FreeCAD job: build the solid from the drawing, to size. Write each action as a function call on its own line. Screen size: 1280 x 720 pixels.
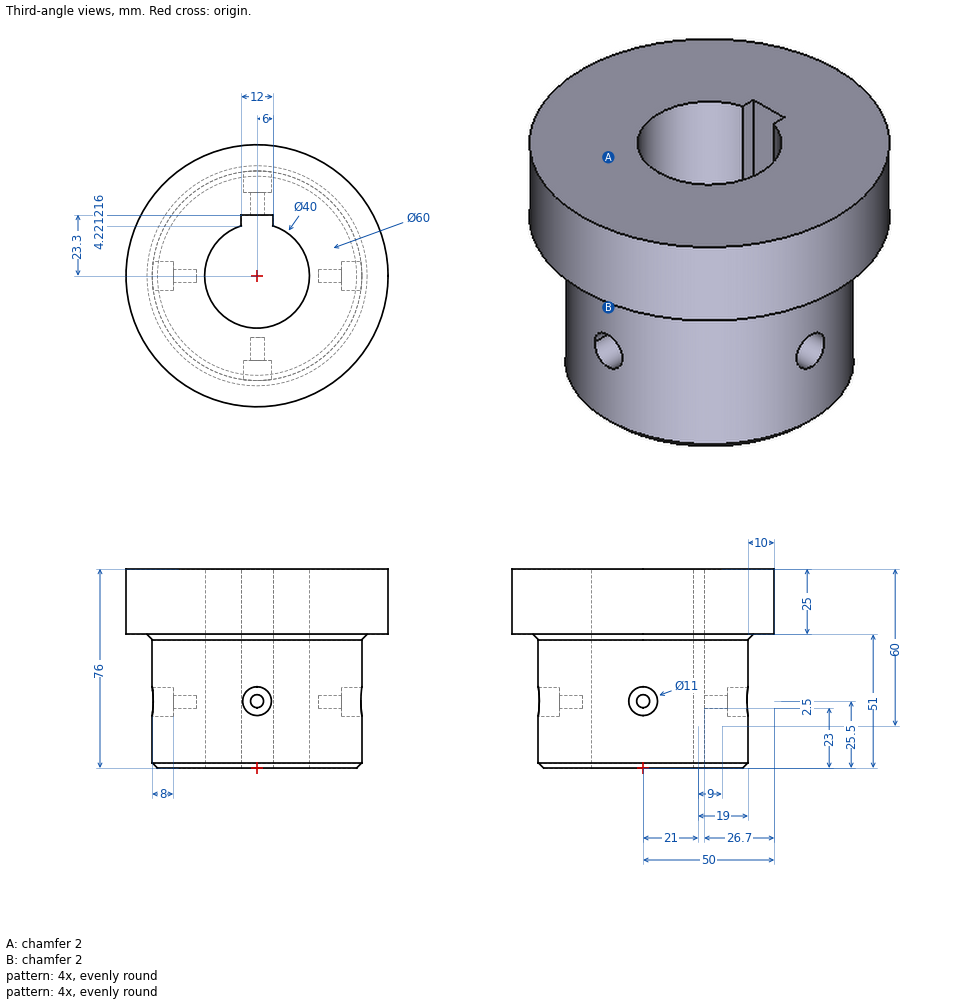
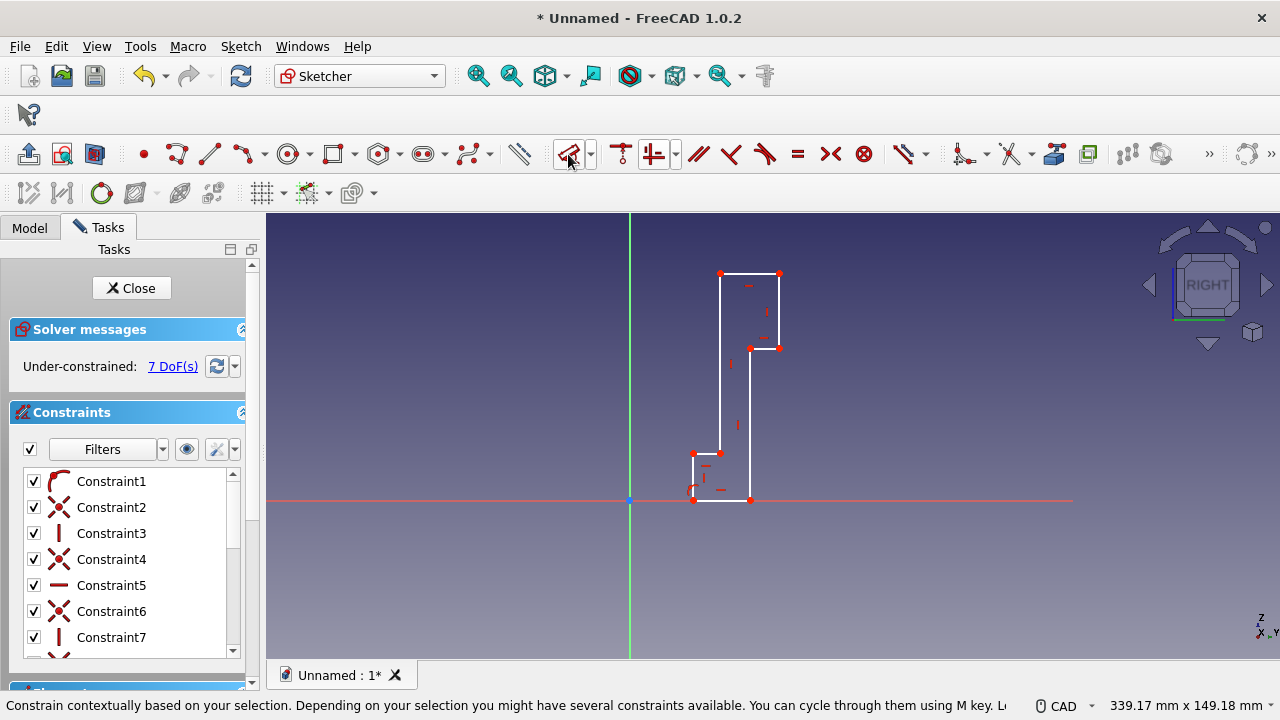
scroll(709, 454, up, 2)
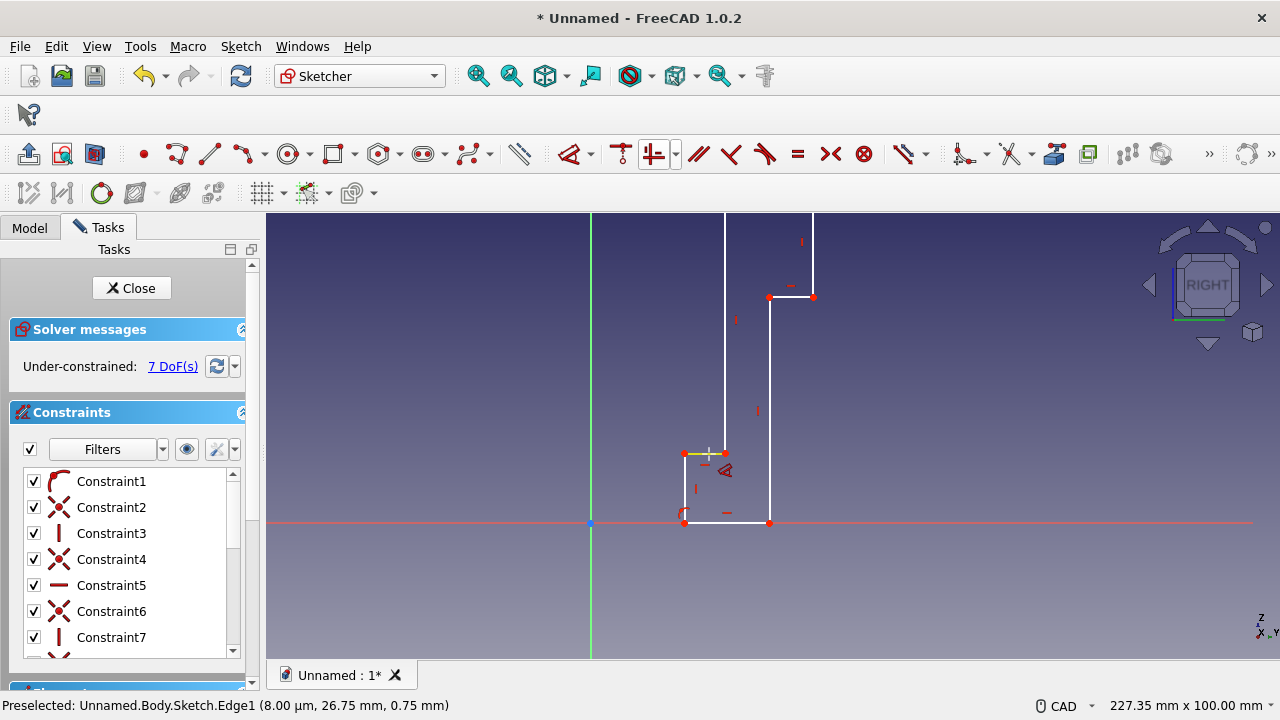
click(709, 454)
click(705, 488)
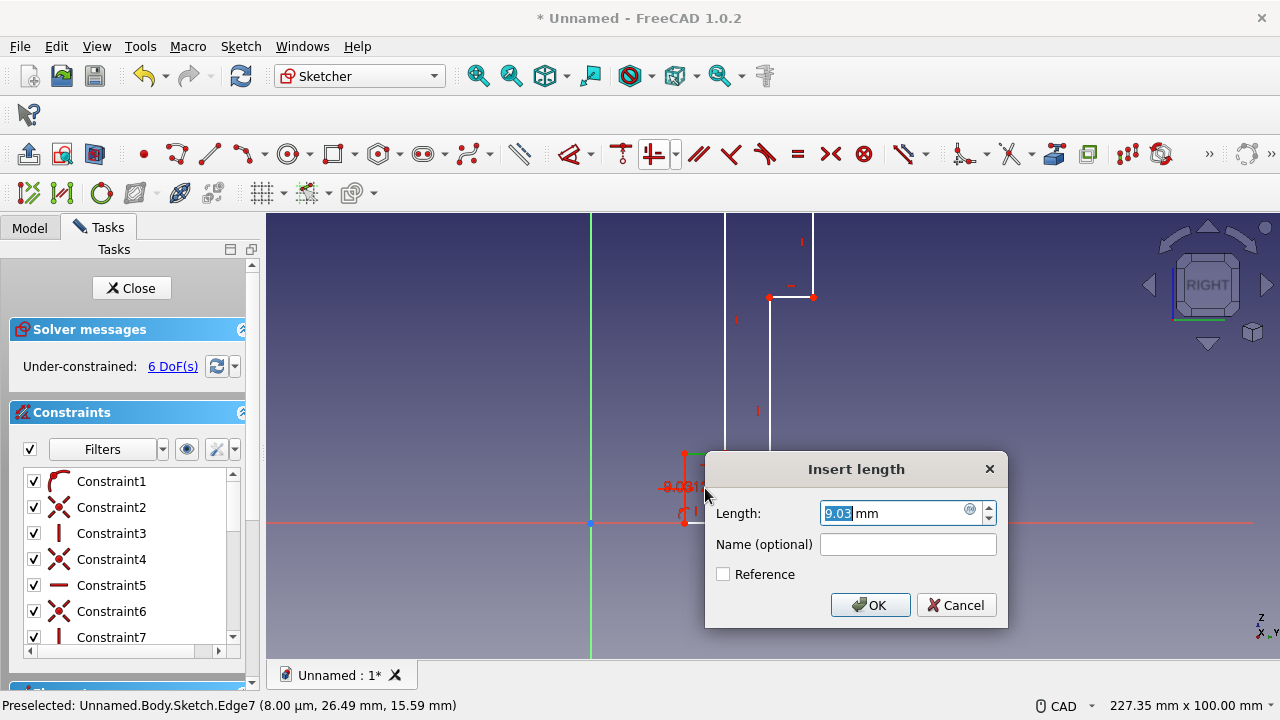
text(9)
key(Return)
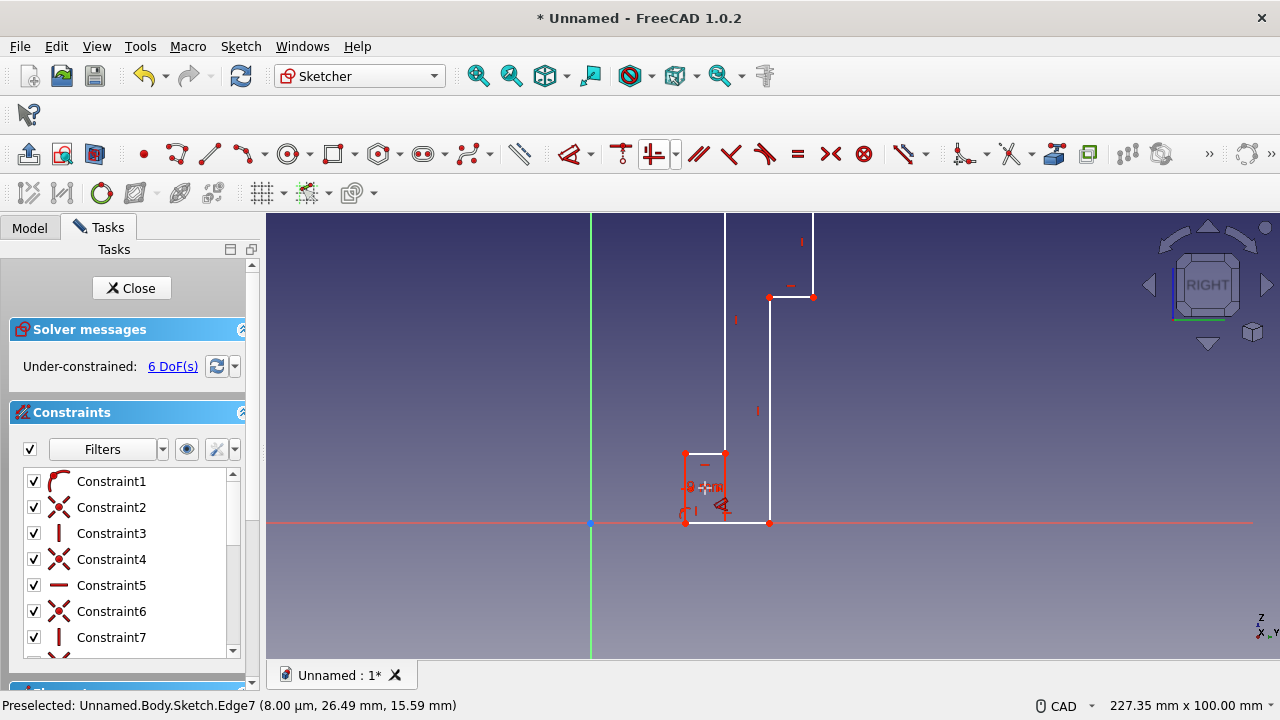
click(711, 523)
click(728, 557)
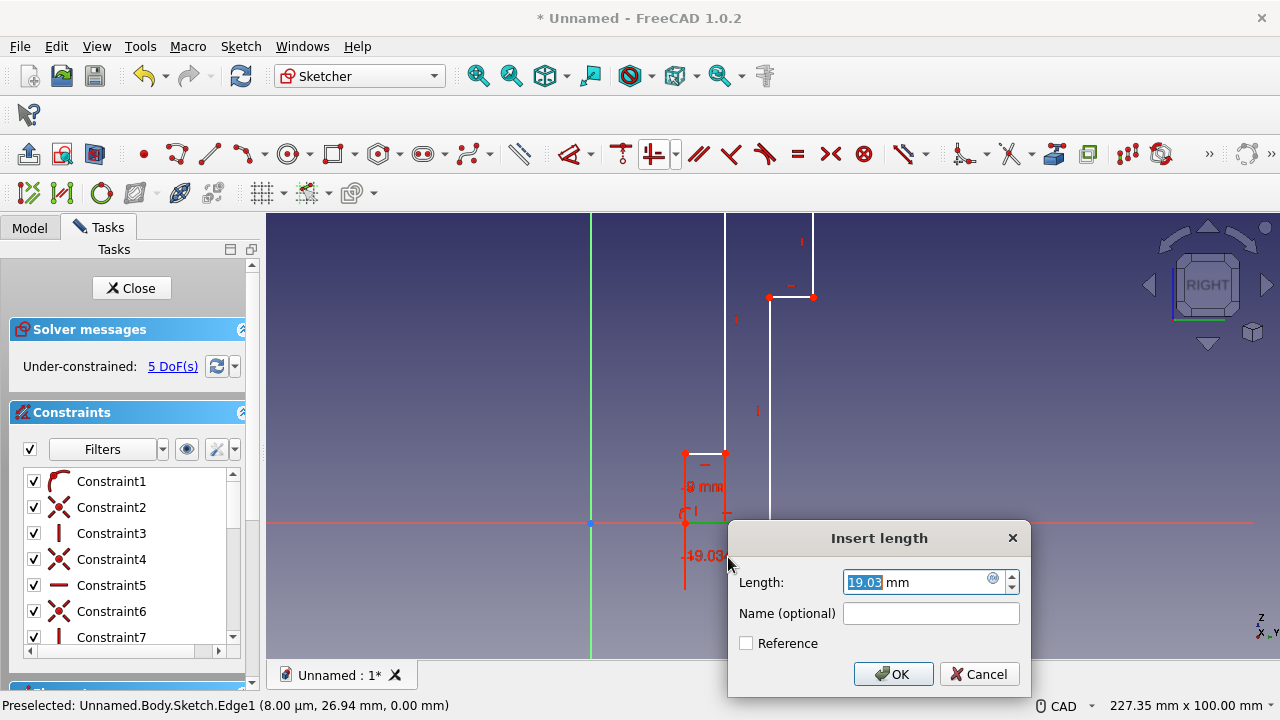
text(19)
key(Return)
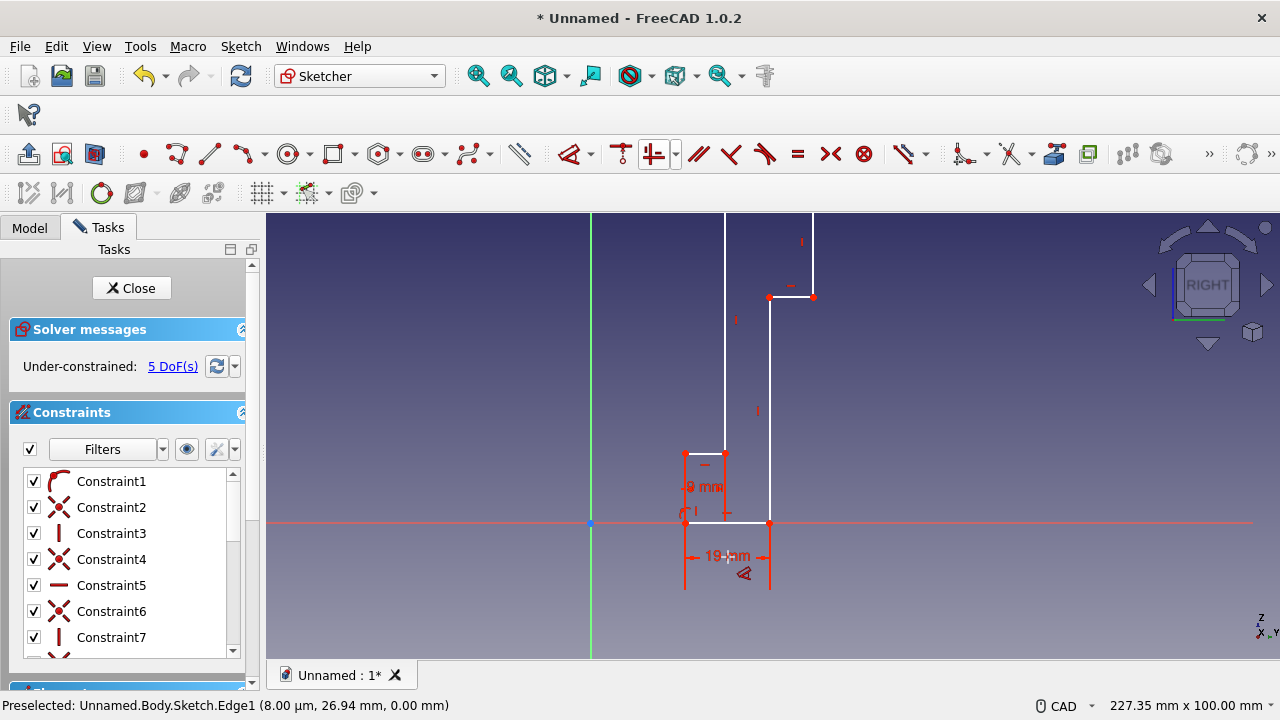
click(770, 455)
click(804, 410)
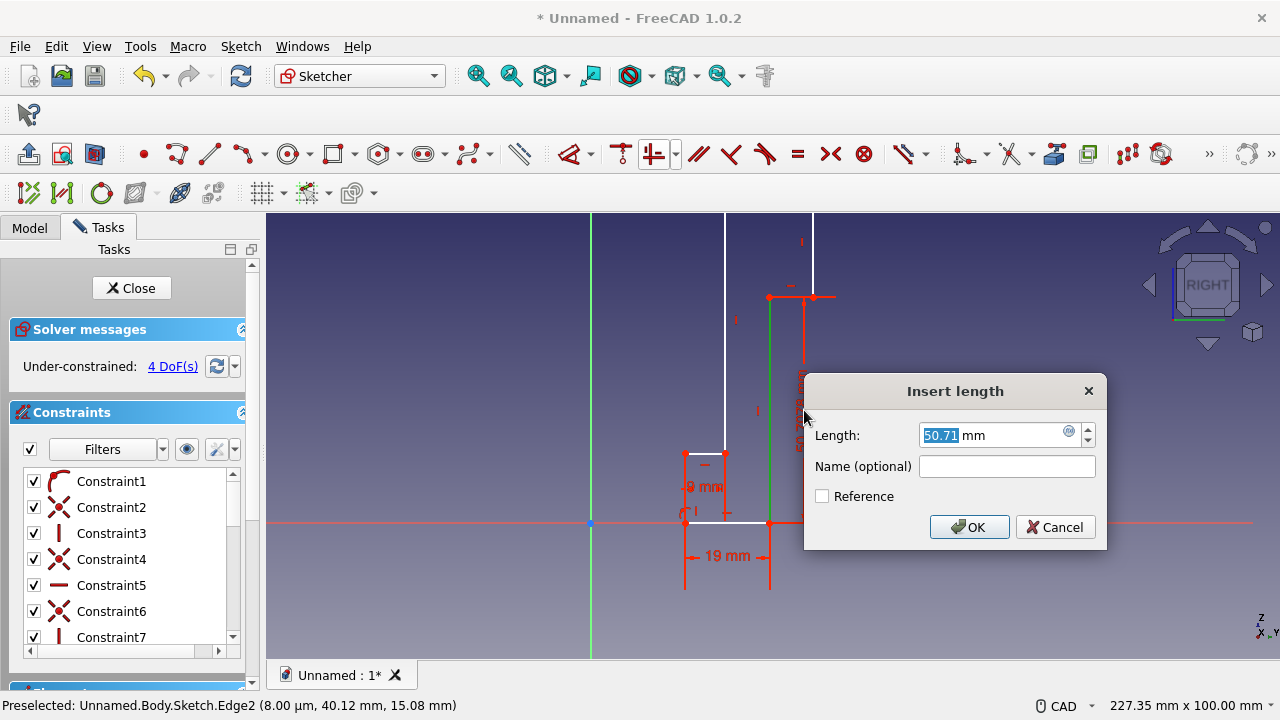
text(51)
key(Return)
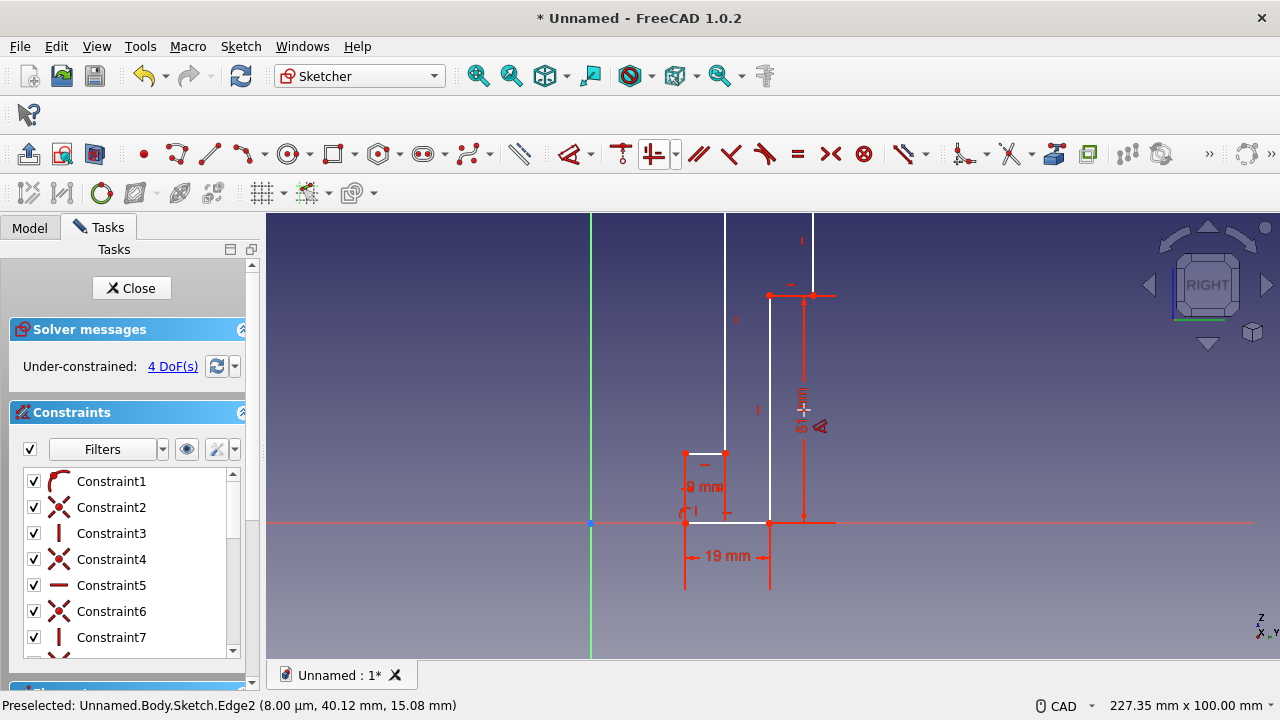
click(783, 296)
click(792, 262)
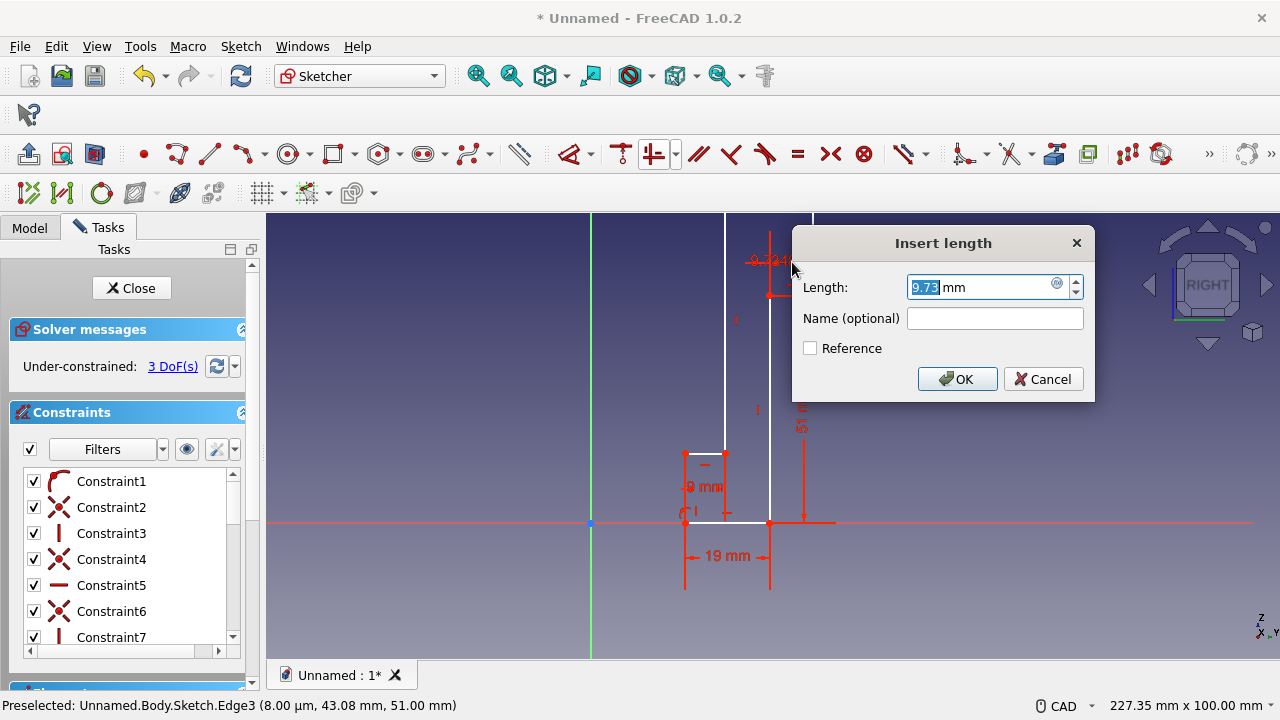
text(10)
key(Return)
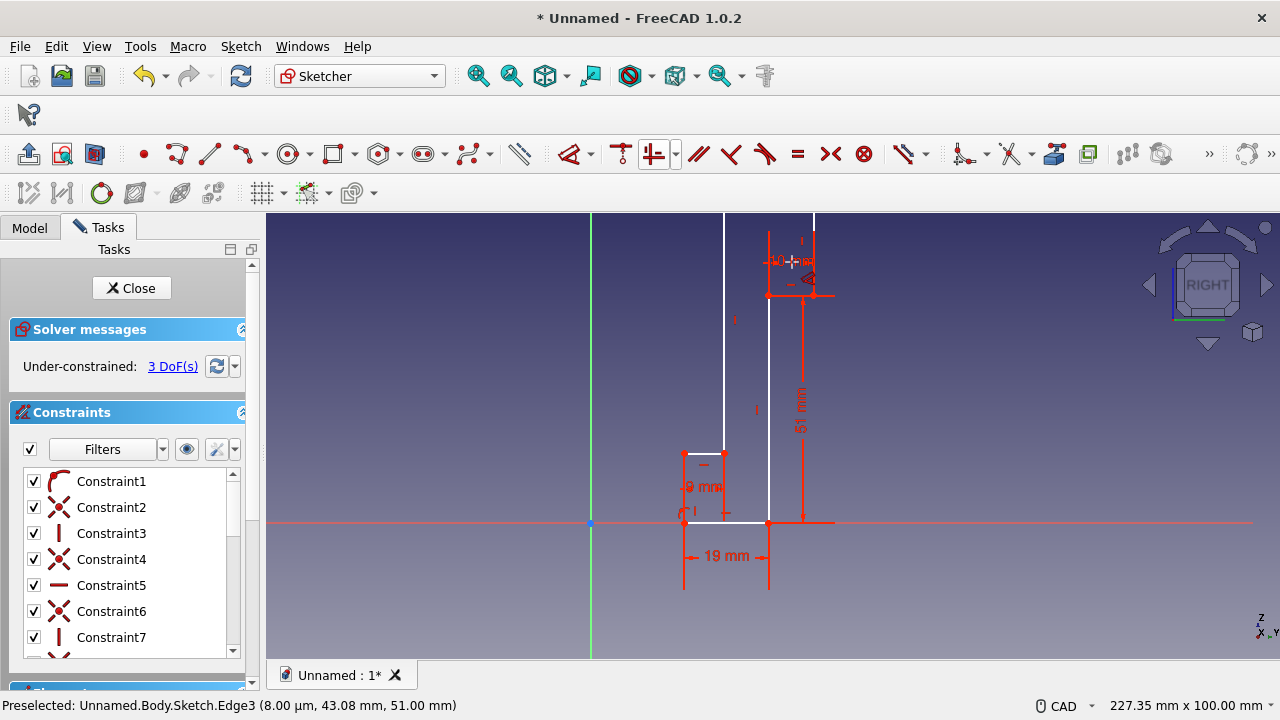
click(814, 263)
click(848, 288)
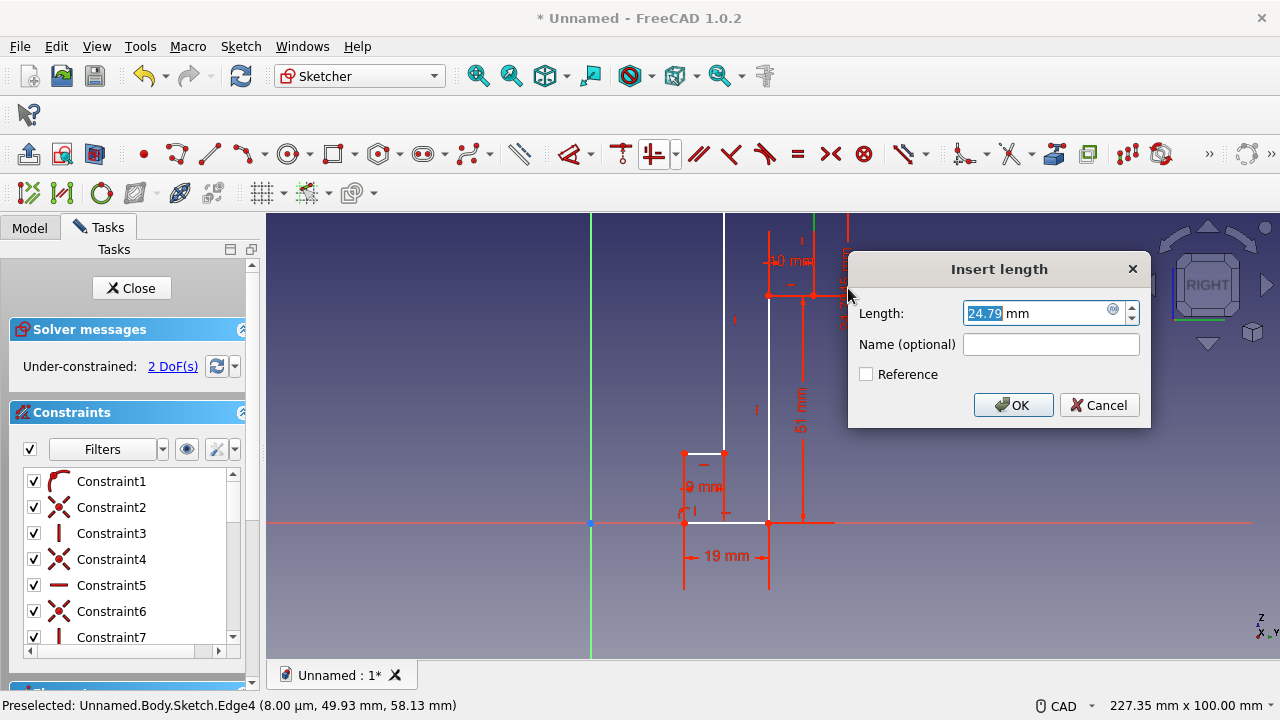
text(25)
key(Return)